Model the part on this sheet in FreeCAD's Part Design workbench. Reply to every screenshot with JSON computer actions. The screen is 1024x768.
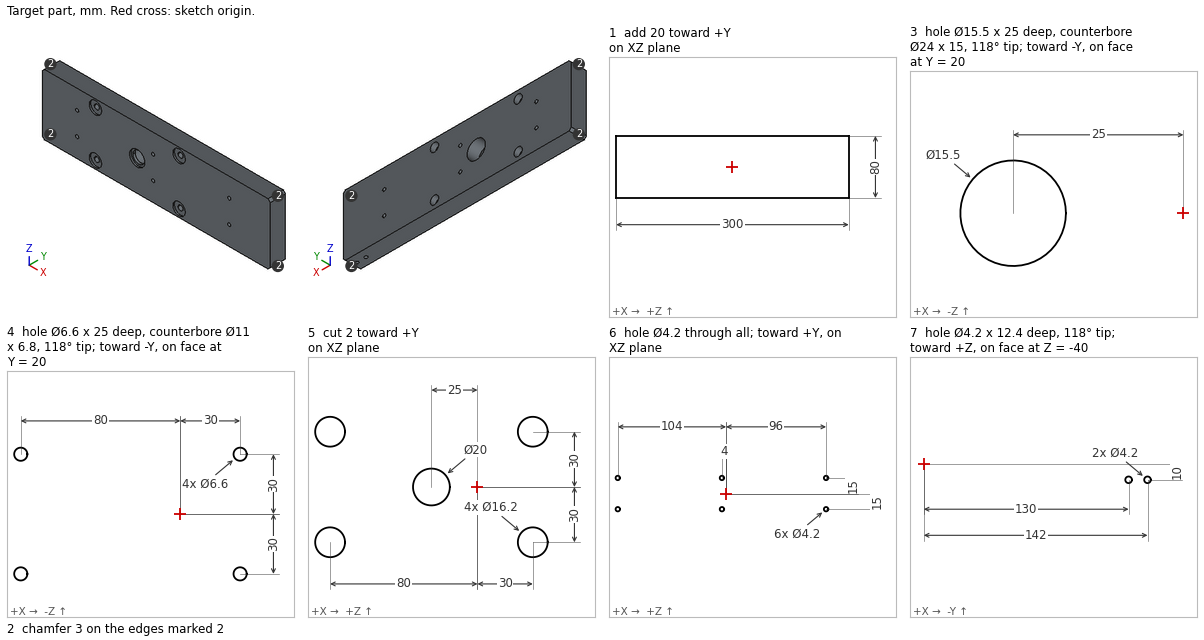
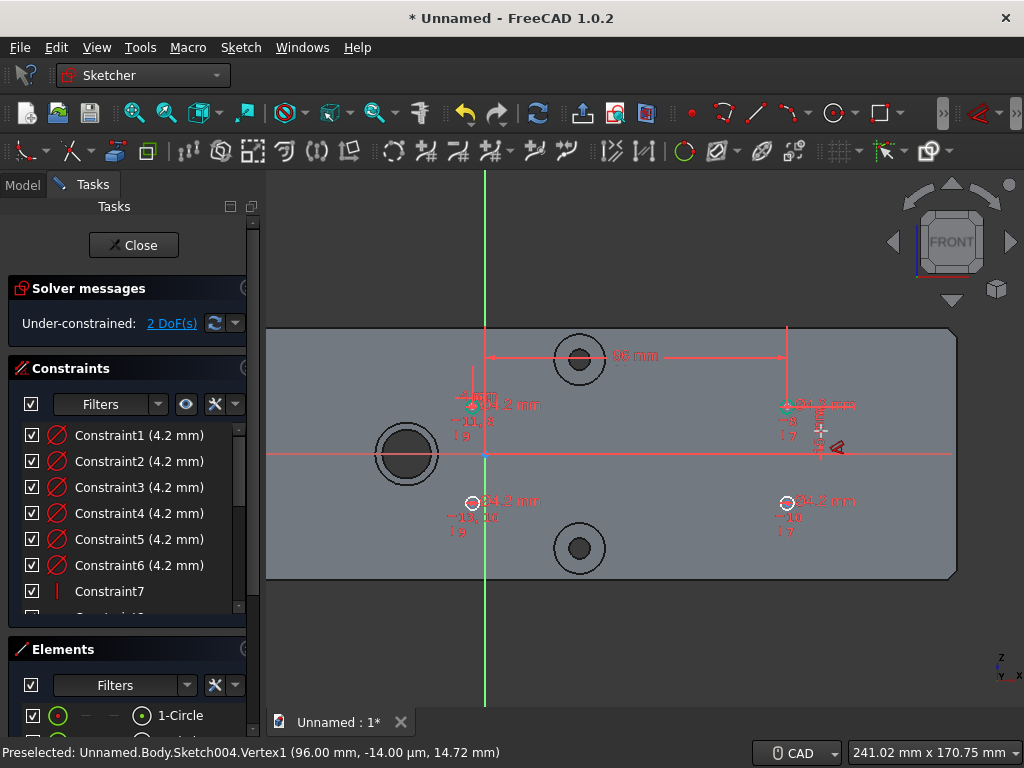
{"action": "left_click", "coordinate": [787, 503]}
{"action": "left_click", "coordinate": [821, 479]}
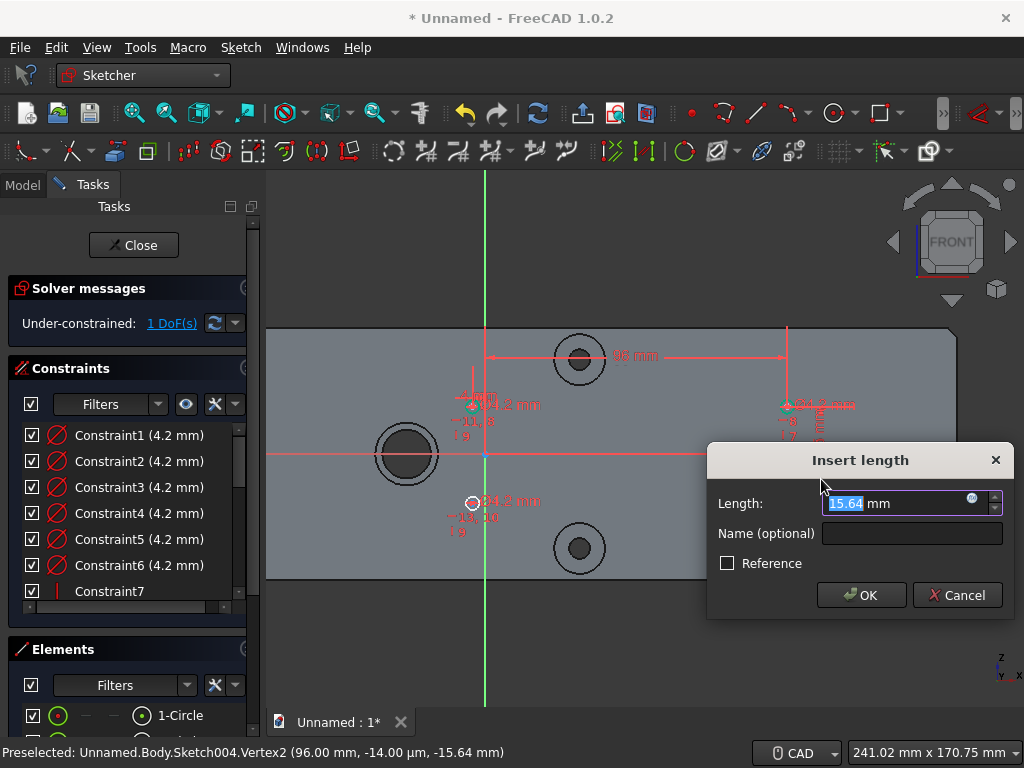
{"action": "type", "text": "15"}
{"action": "key", "text": "Return"}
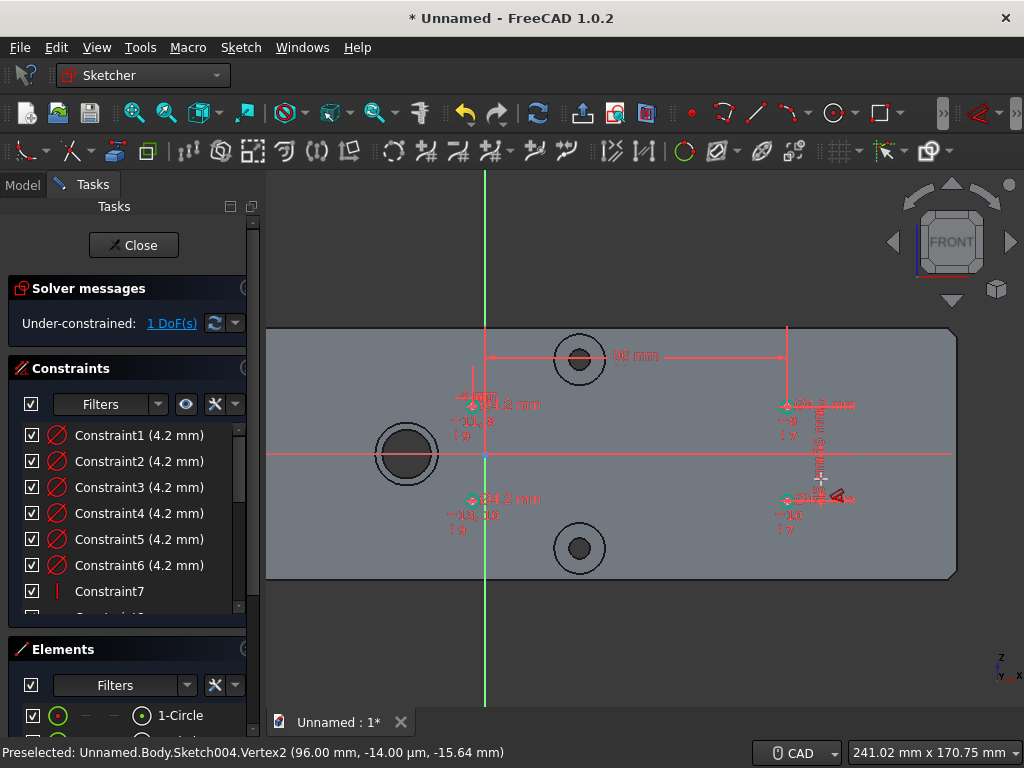
{"action": "scroll", "coordinate": [788, 407], "scroll_direction": "down", "scroll_amount": 2}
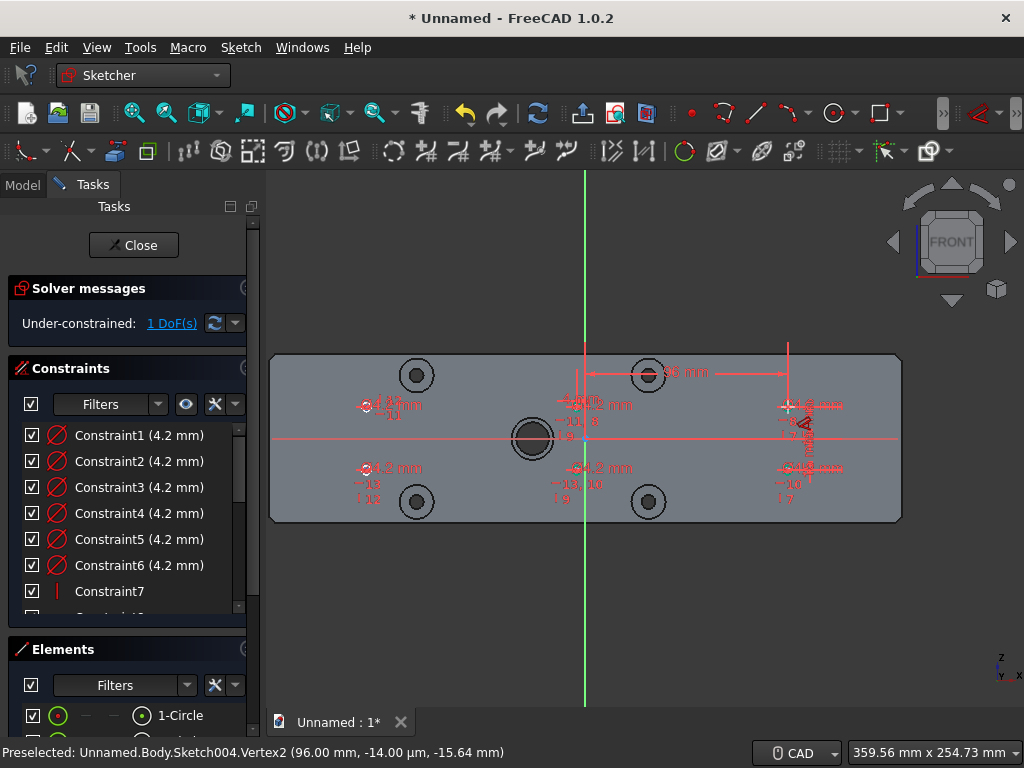
{"action": "left_click", "coordinate": [366, 407]}
{"action": "left_click", "coordinate": [476, 373]}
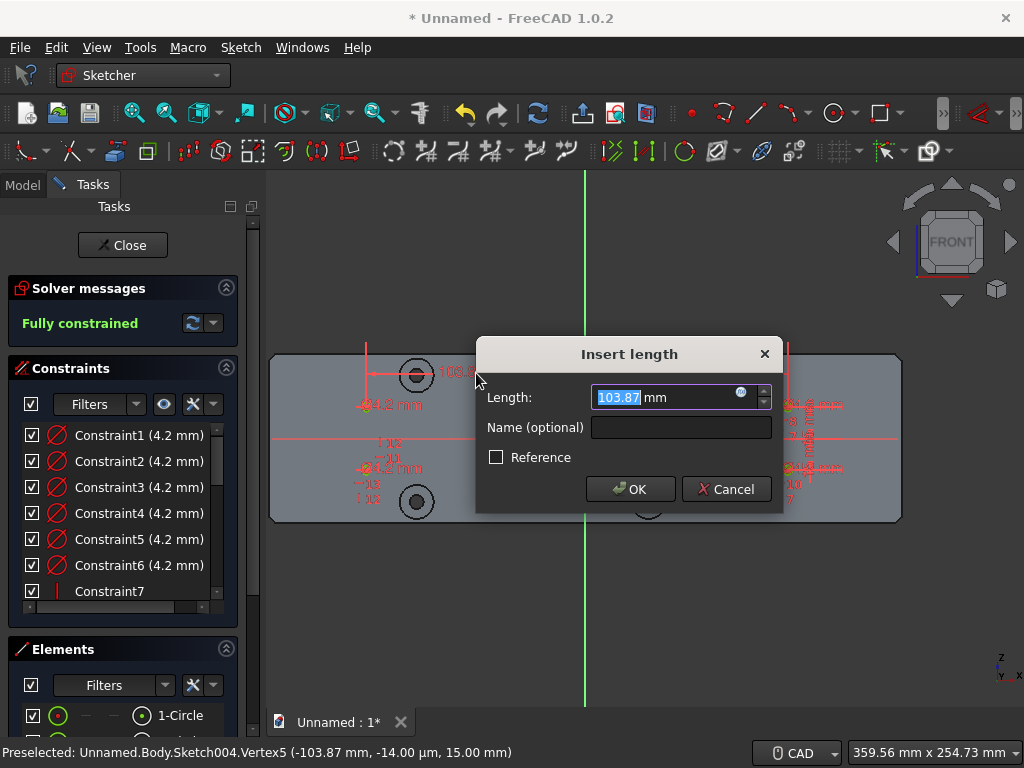
{"action": "type", "text": "104"}
{"action": "key", "text": "Return"}
{"action": "key", "text": "Escape"}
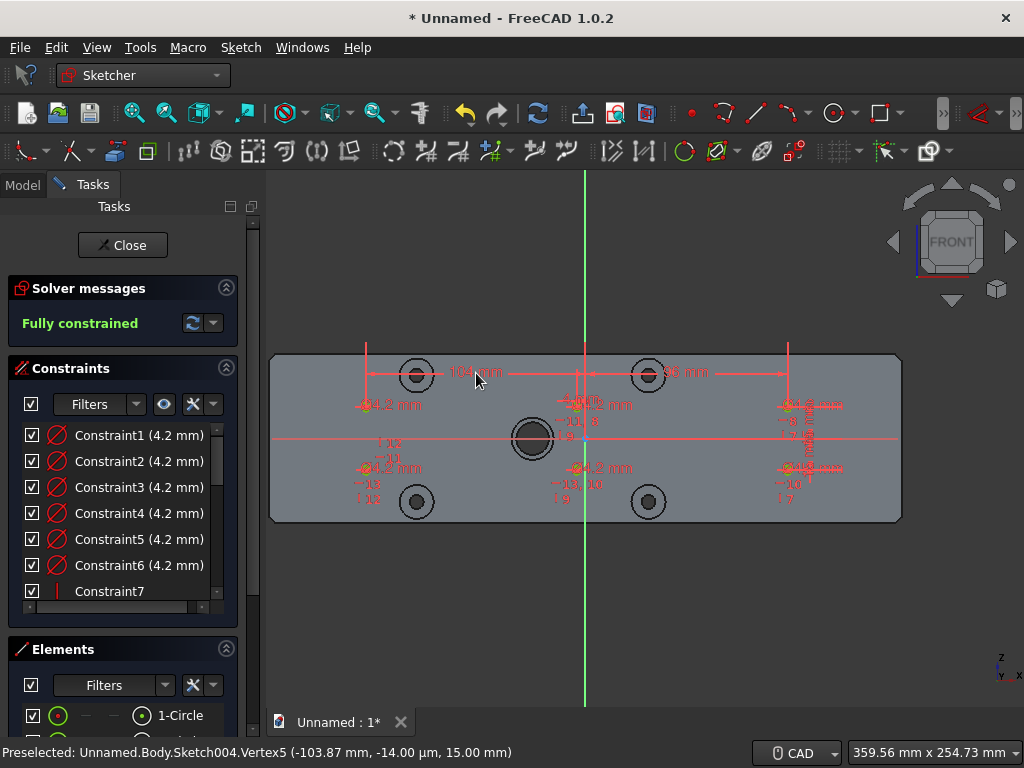
{"action": "left_click", "coordinate": [123, 245]}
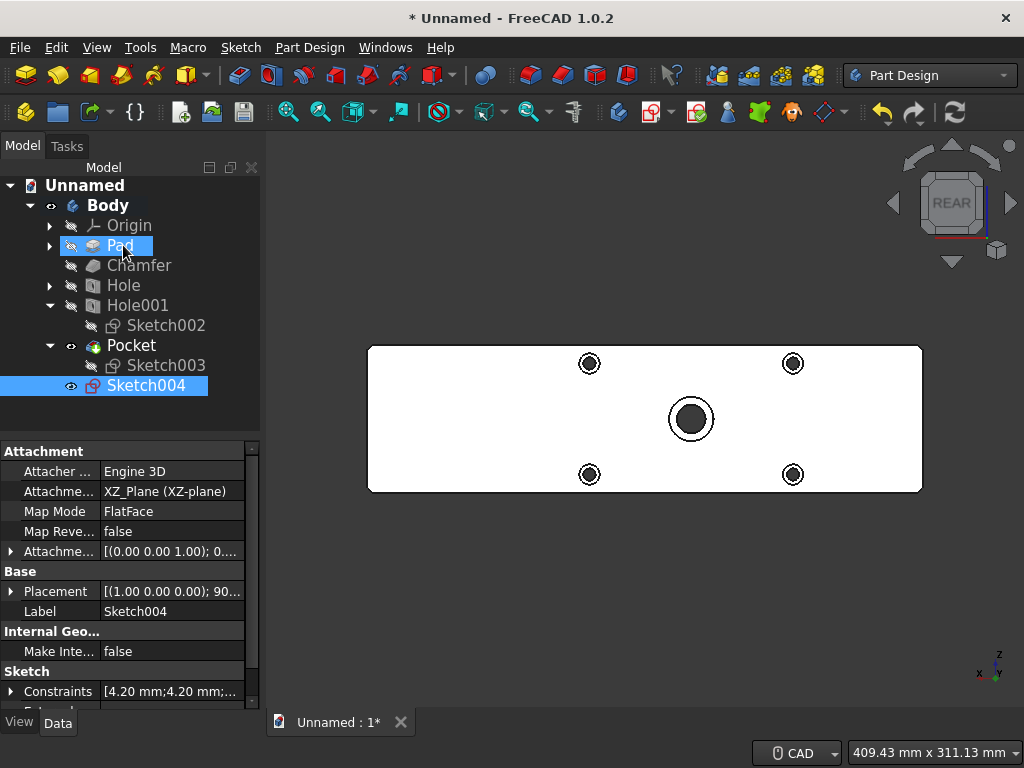
{"action": "left_click", "coordinate": [272, 76]}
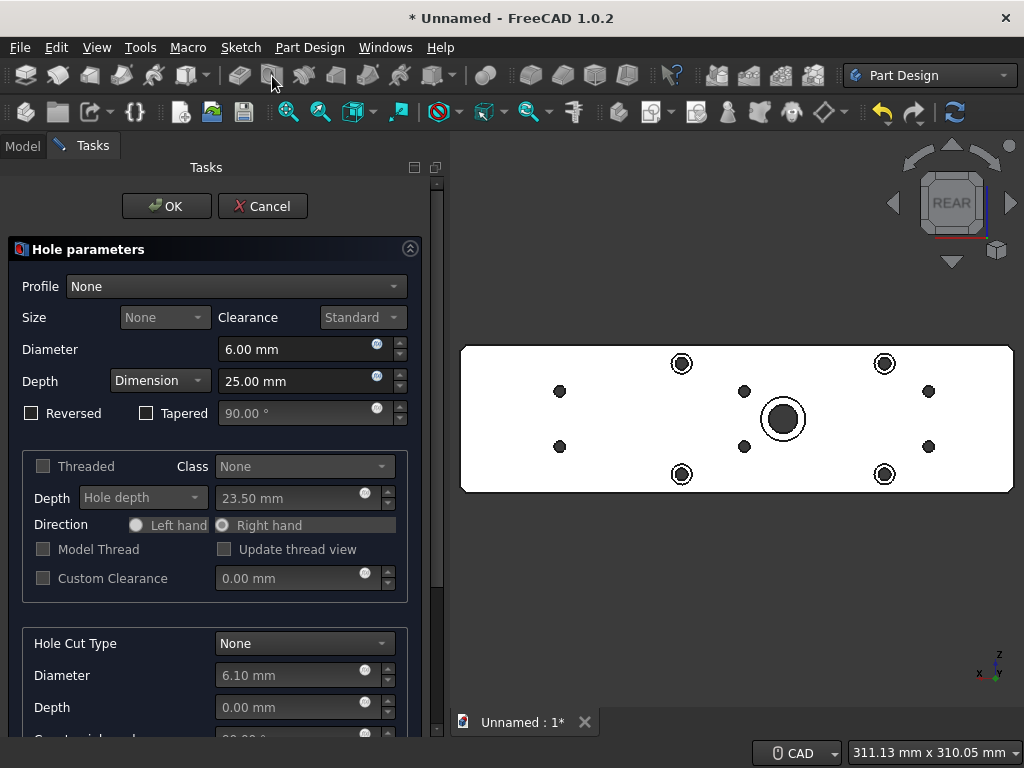
{"action": "triple_click", "coordinate": [305, 349]}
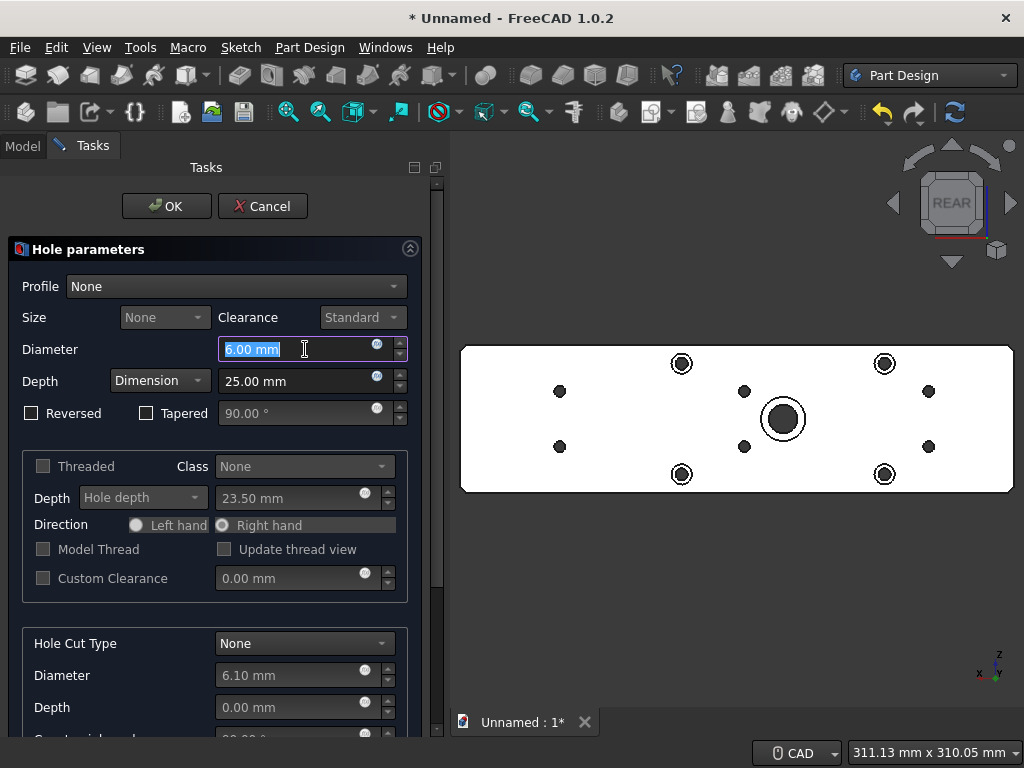
{"action": "type", "text": "4.2"}
{"action": "key", "text": "Tab"}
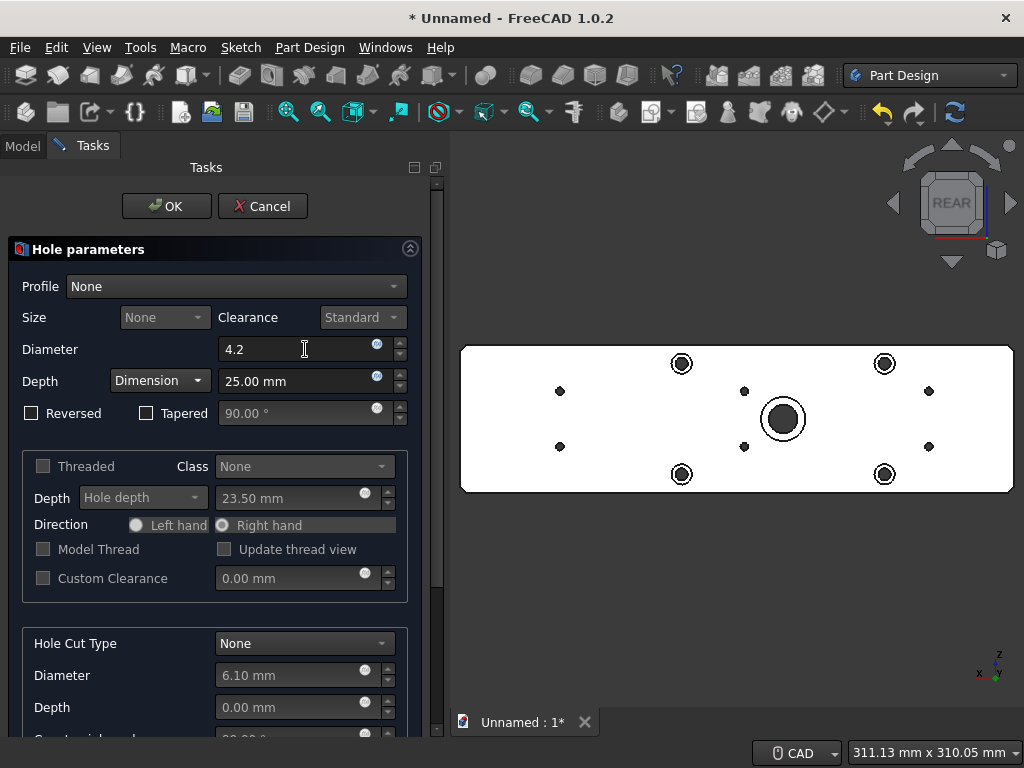
{"action": "left_click", "coordinate": [161, 380]}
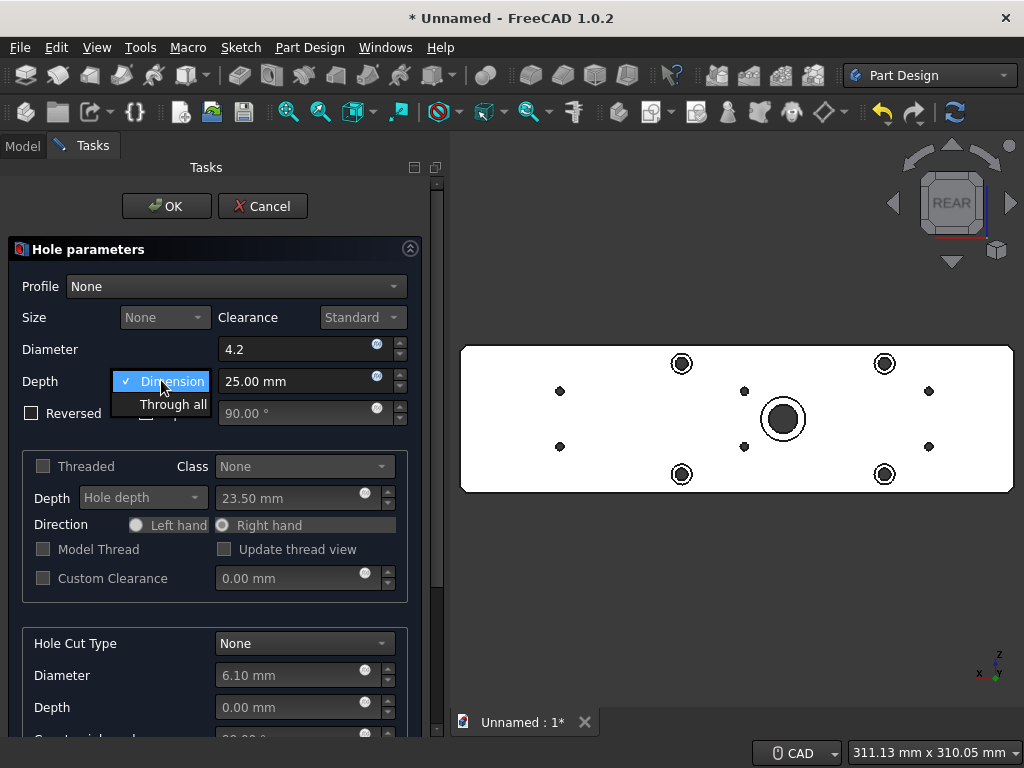
{"action": "left_click", "coordinate": [160, 404]}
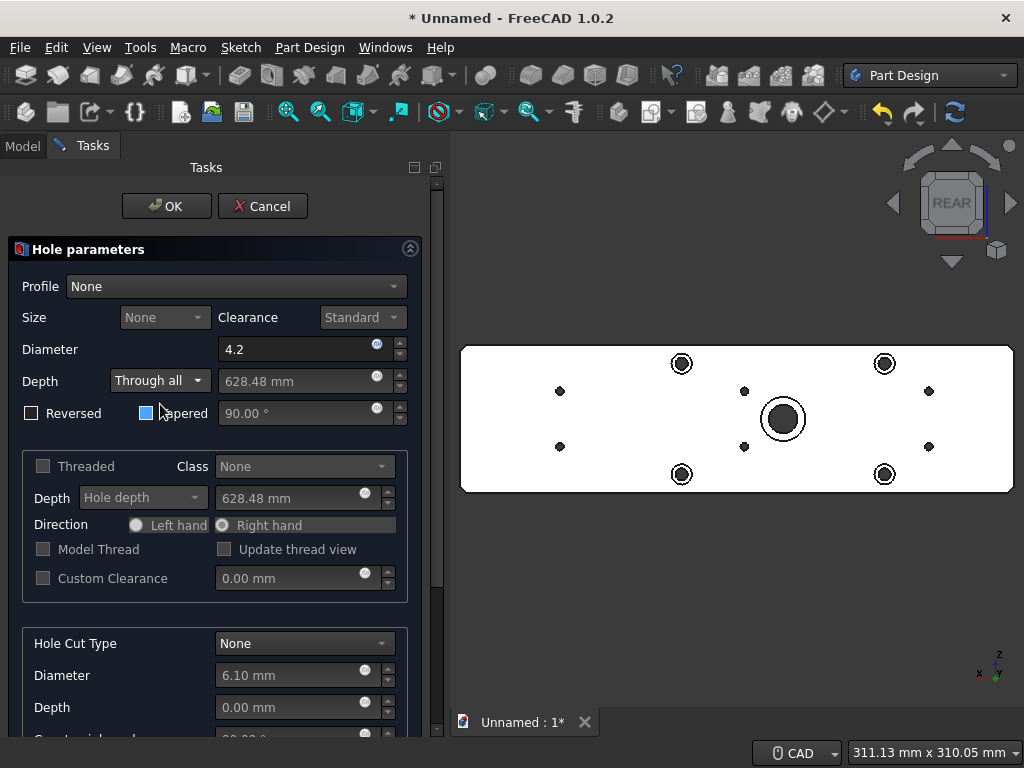
{"action": "left_click", "coordinate": [167, 206]}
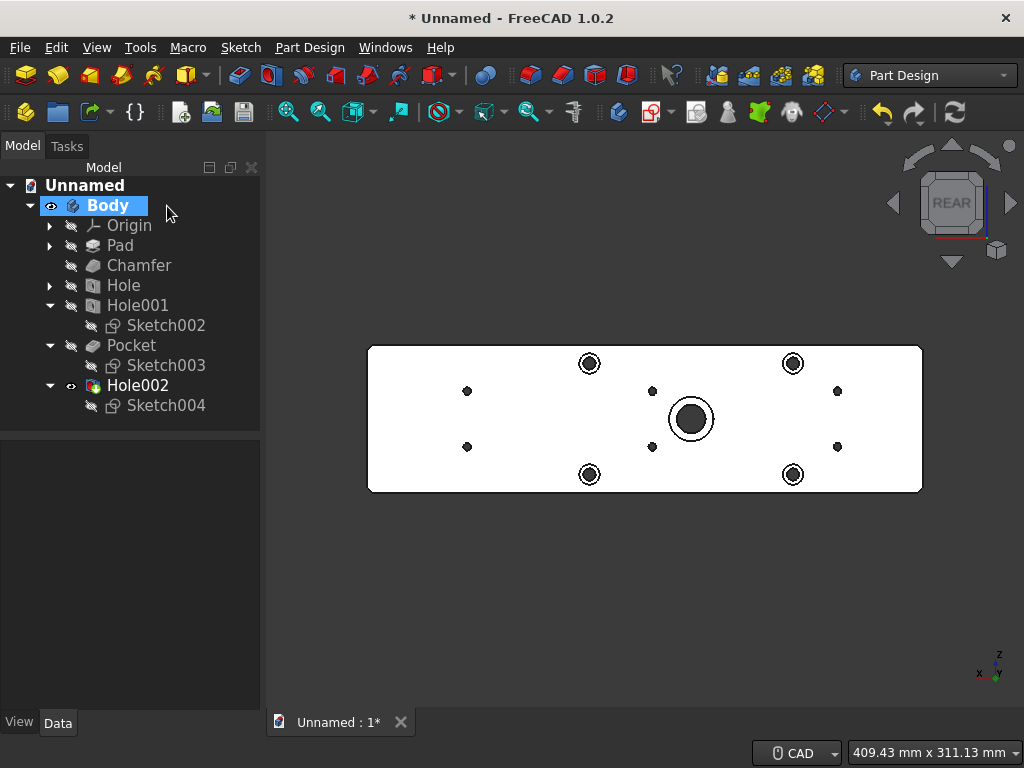
{"action": "key", "text": "5"}